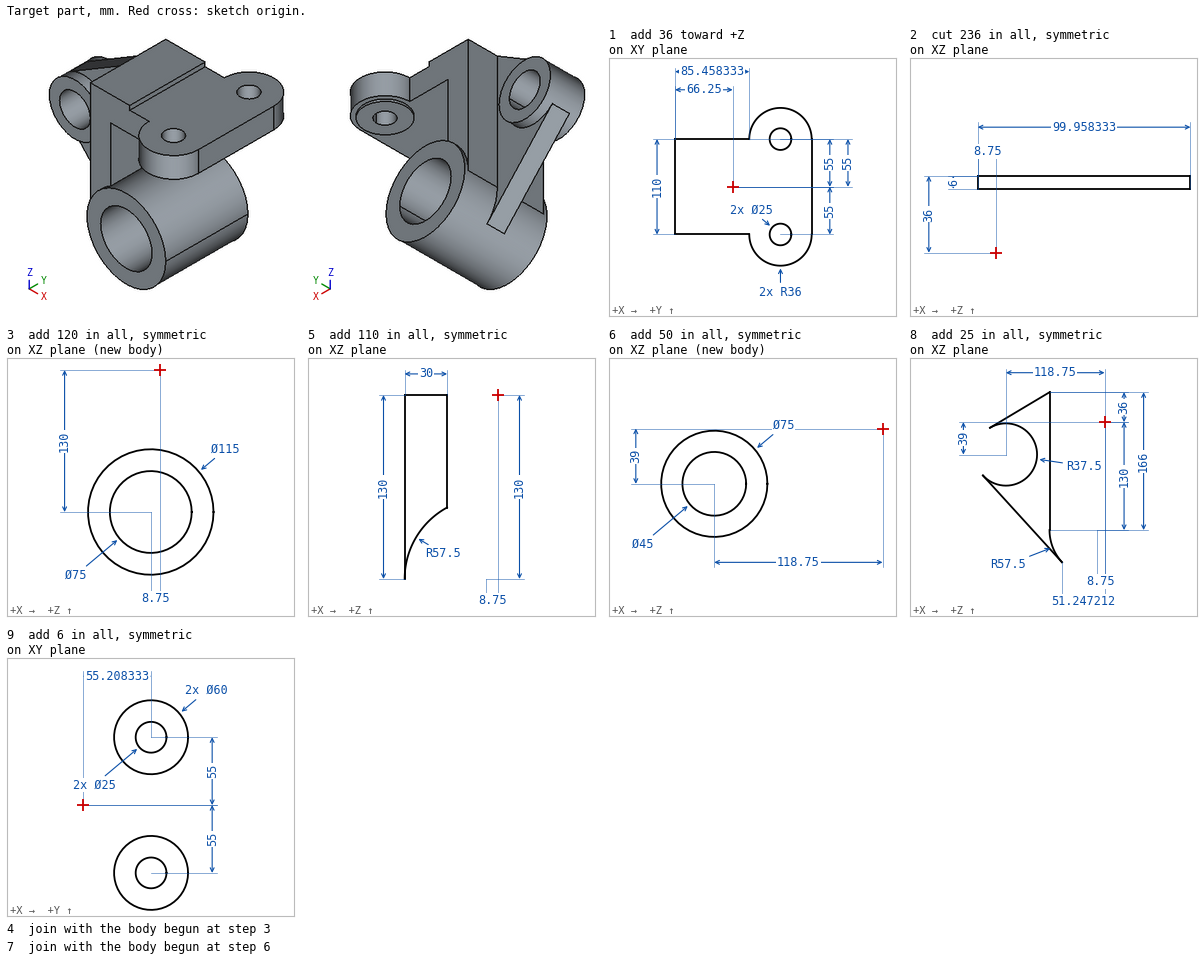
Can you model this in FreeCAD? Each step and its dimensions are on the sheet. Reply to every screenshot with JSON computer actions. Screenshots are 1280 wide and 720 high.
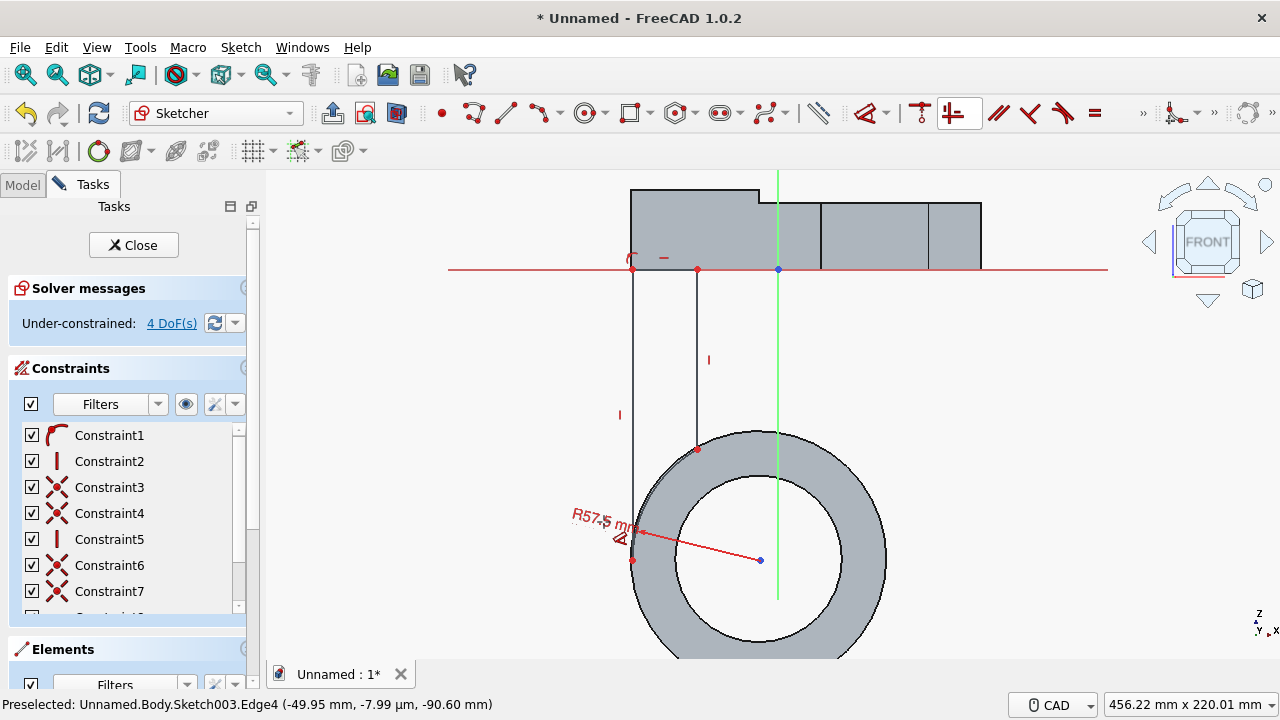
{"action": "left_click", "coordinate": [652, 270]}
{"action": "left_click", "coordinate": [665, 236]}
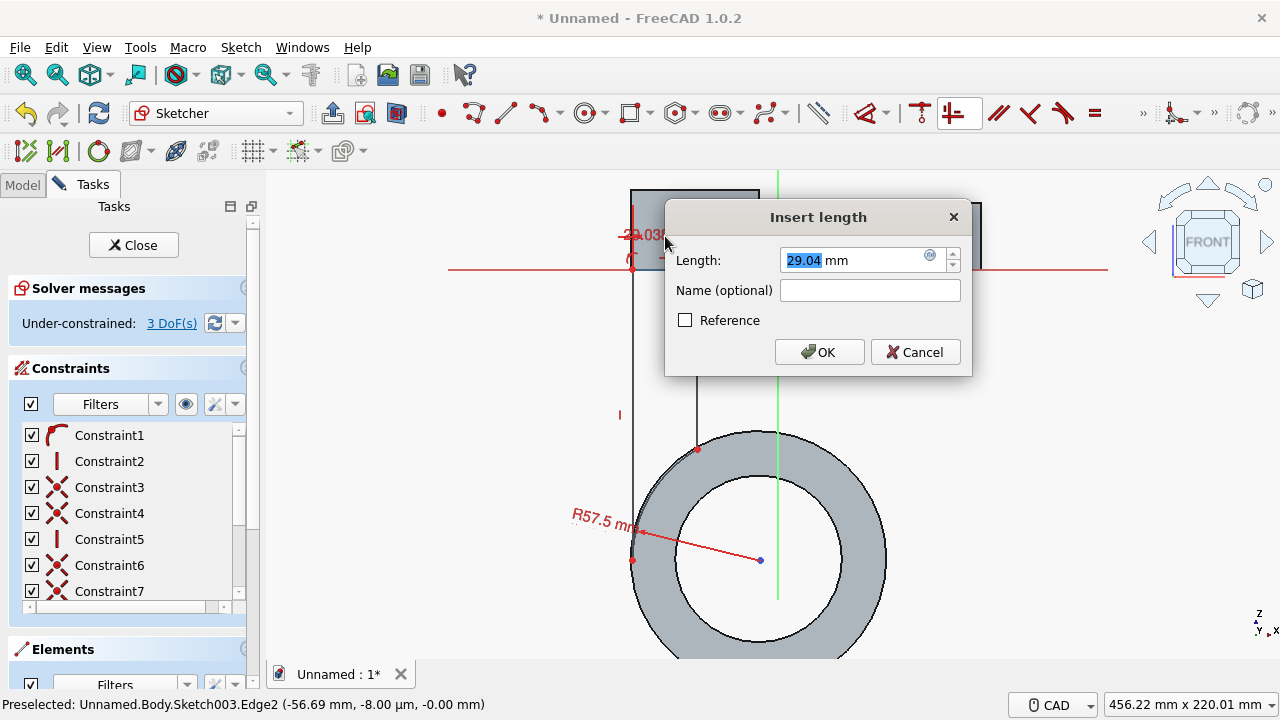
{"action": "type", "text": "30"}
{"action": "key", "text": "Return"}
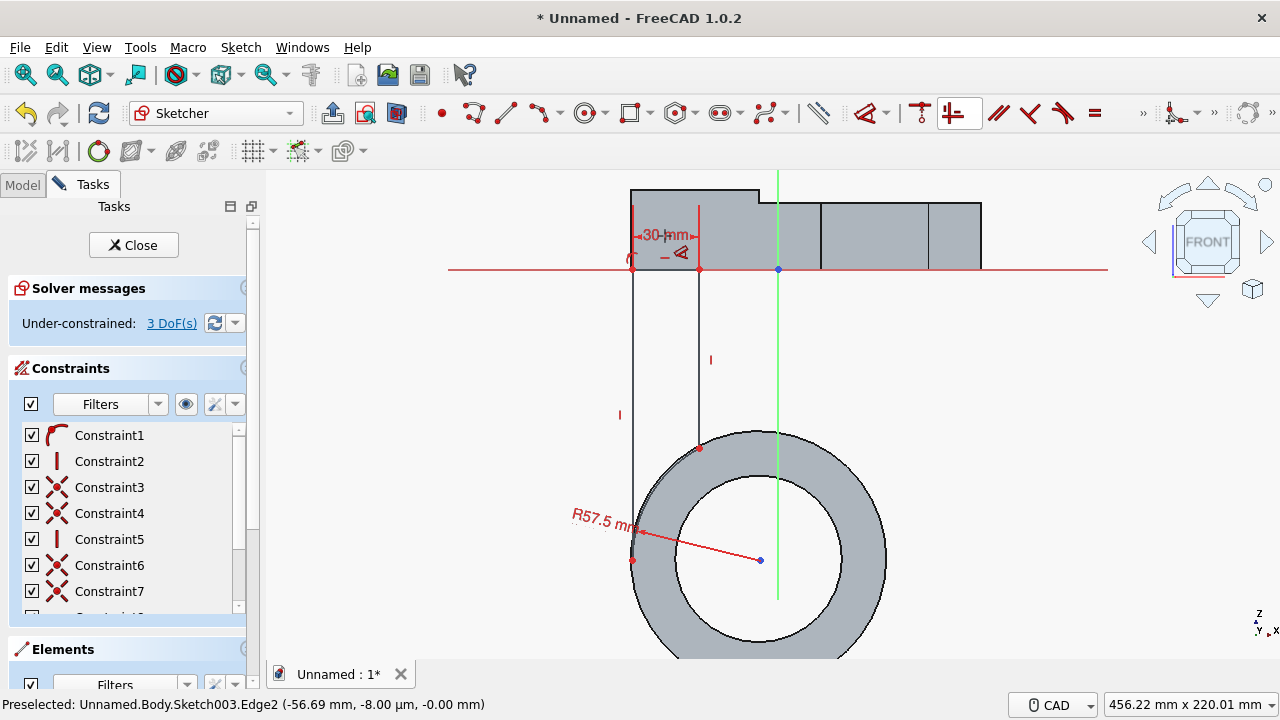
{"action": "left_click", "coordinate": [633, 473]}
{"action": "left_click", "coordinate": [599, 415]}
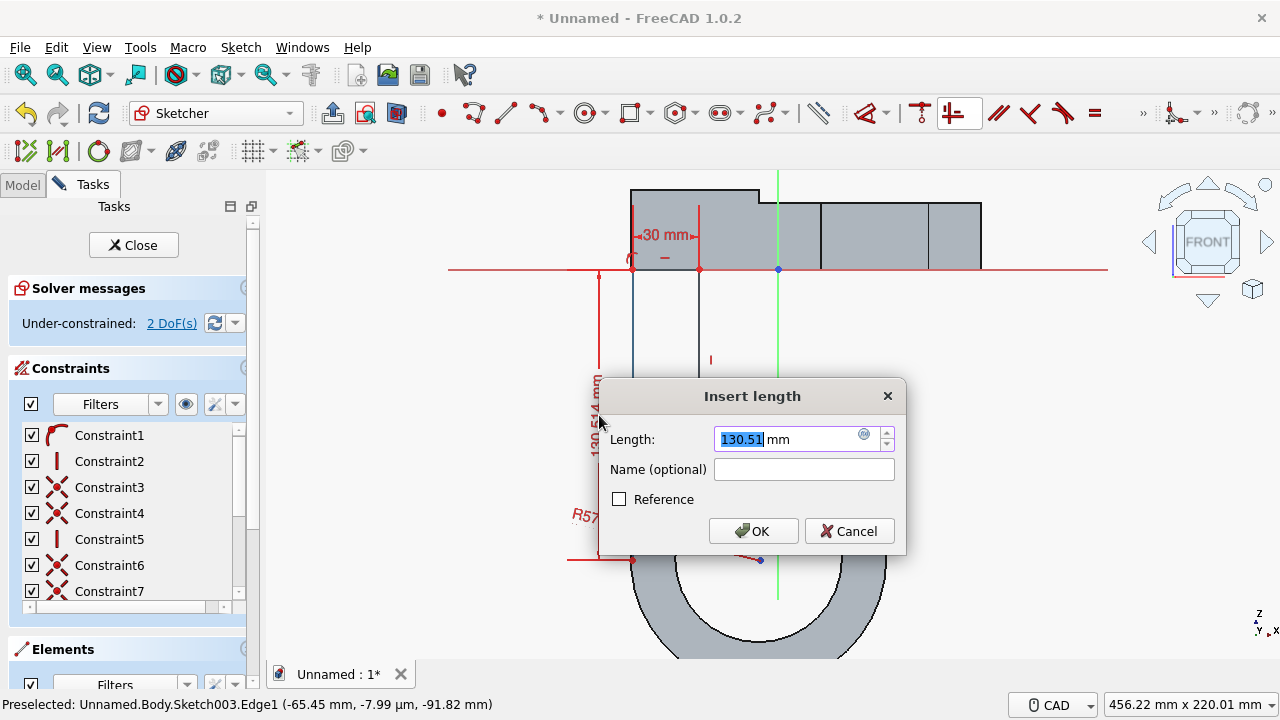
{"action": "type", "text": "130"}
{"action": "key", "text": "Return"}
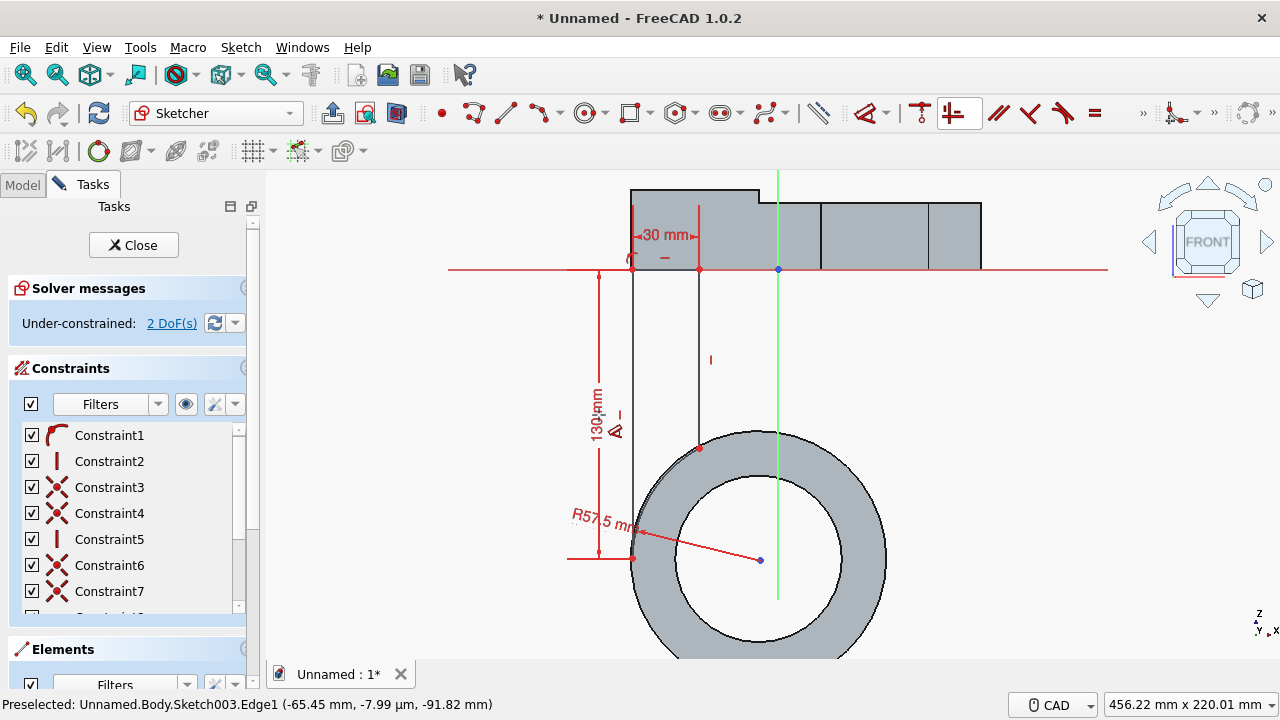
{"action": "left_click", "coordinate": [760, 561]}
{"action": "left_click", "coordinate": [812, 415]}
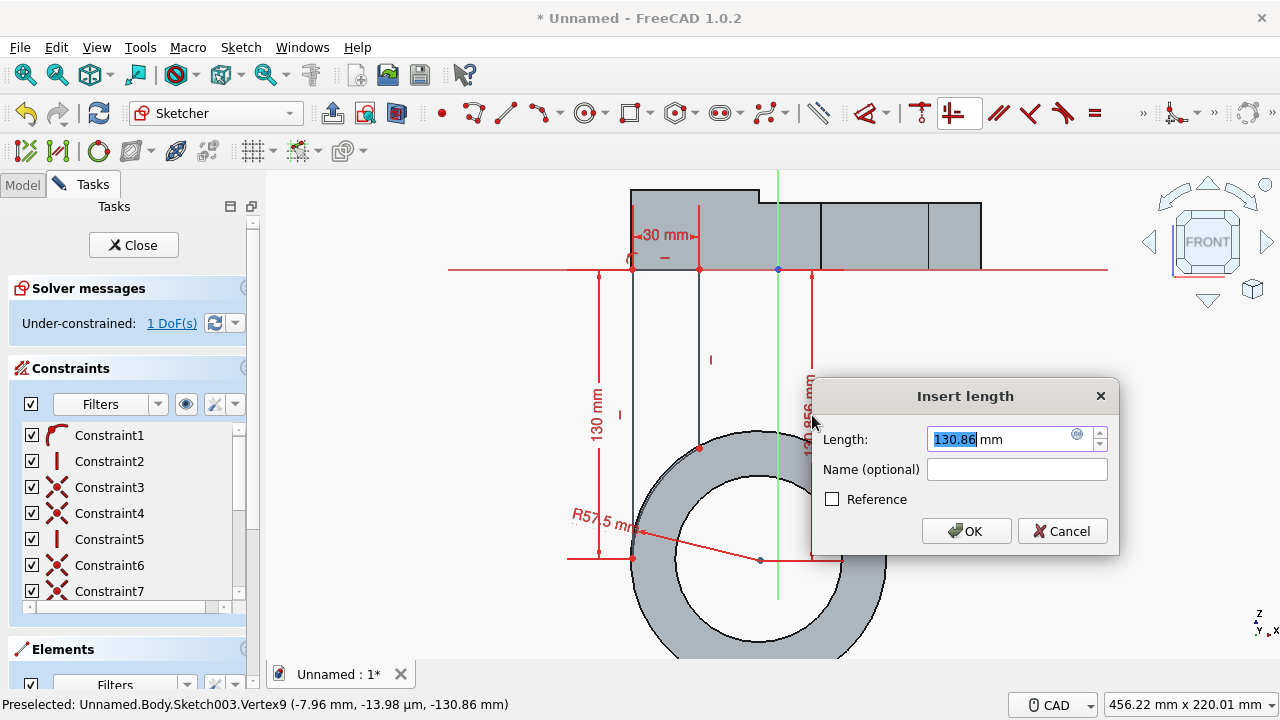
{"action": "type", "text": "130"}
{"action": "key", "text": "Return"}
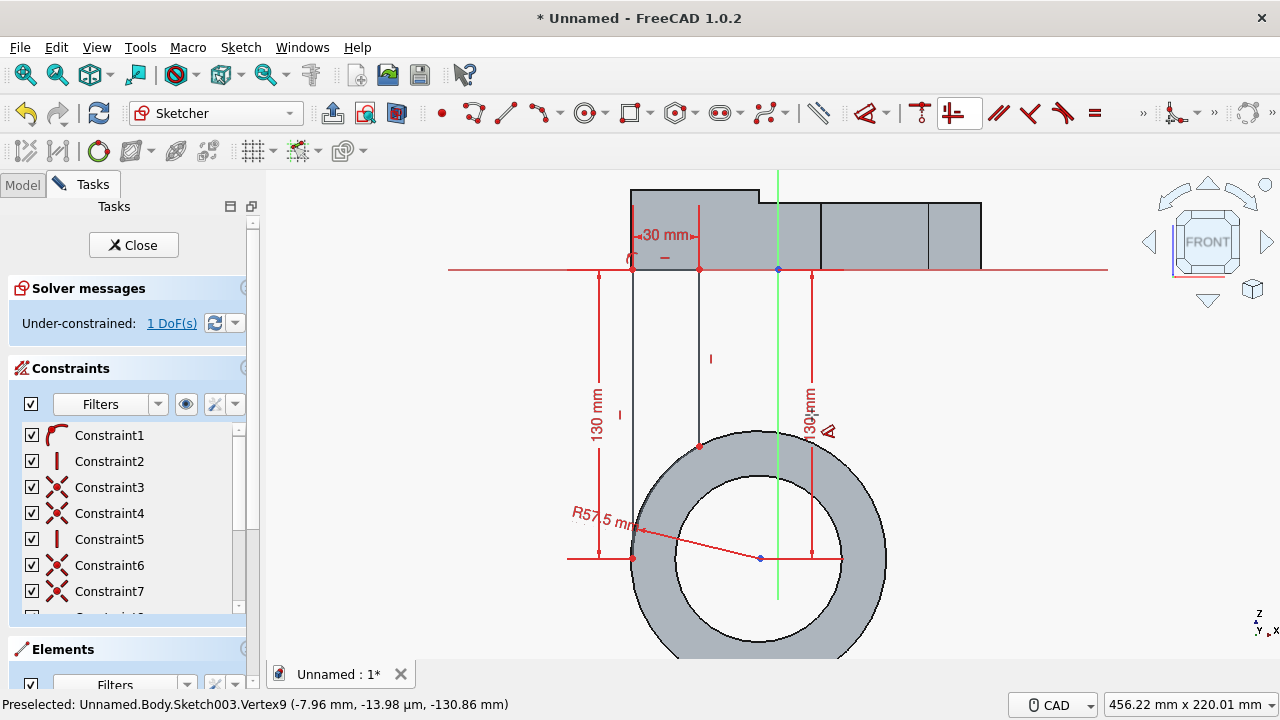
{"action": "scroll", "coordinate": [760, 559], "scroll_direction": "up", "scroll_amount": 4}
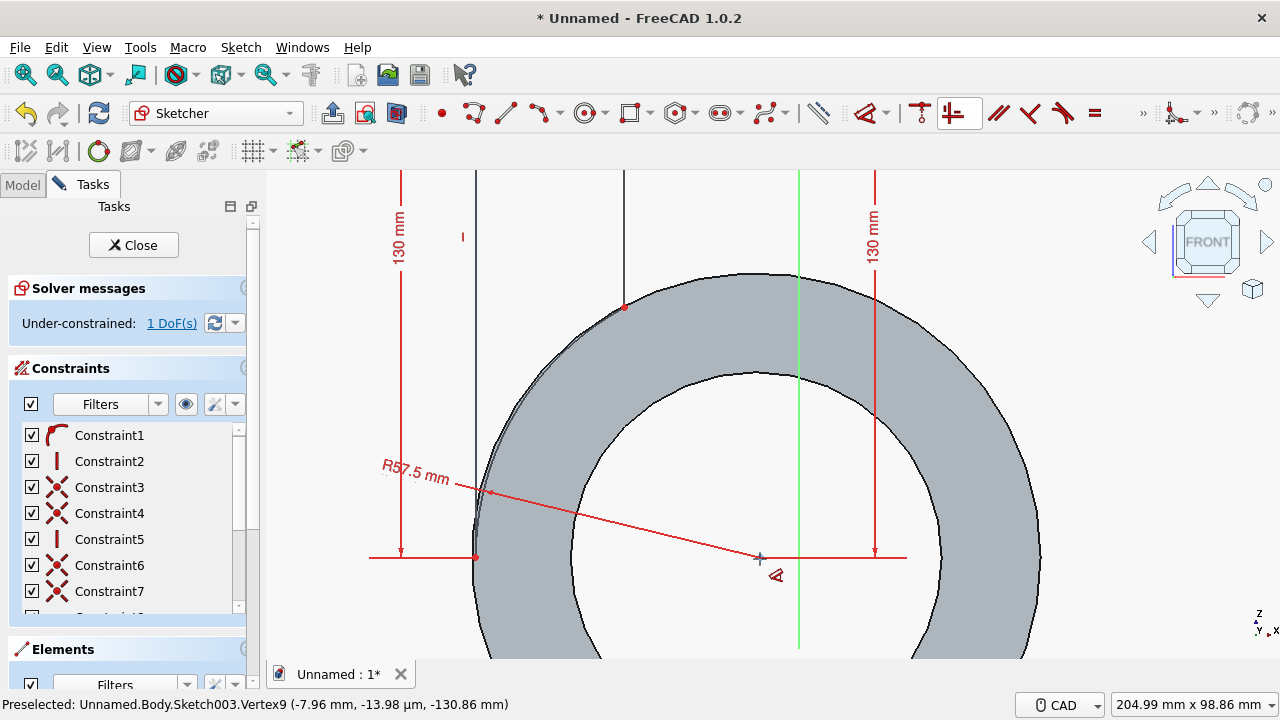
{"action": "left_click", "coordinate": [760, 558]}
{"action": "left_click", "coordinate": [780, 592]}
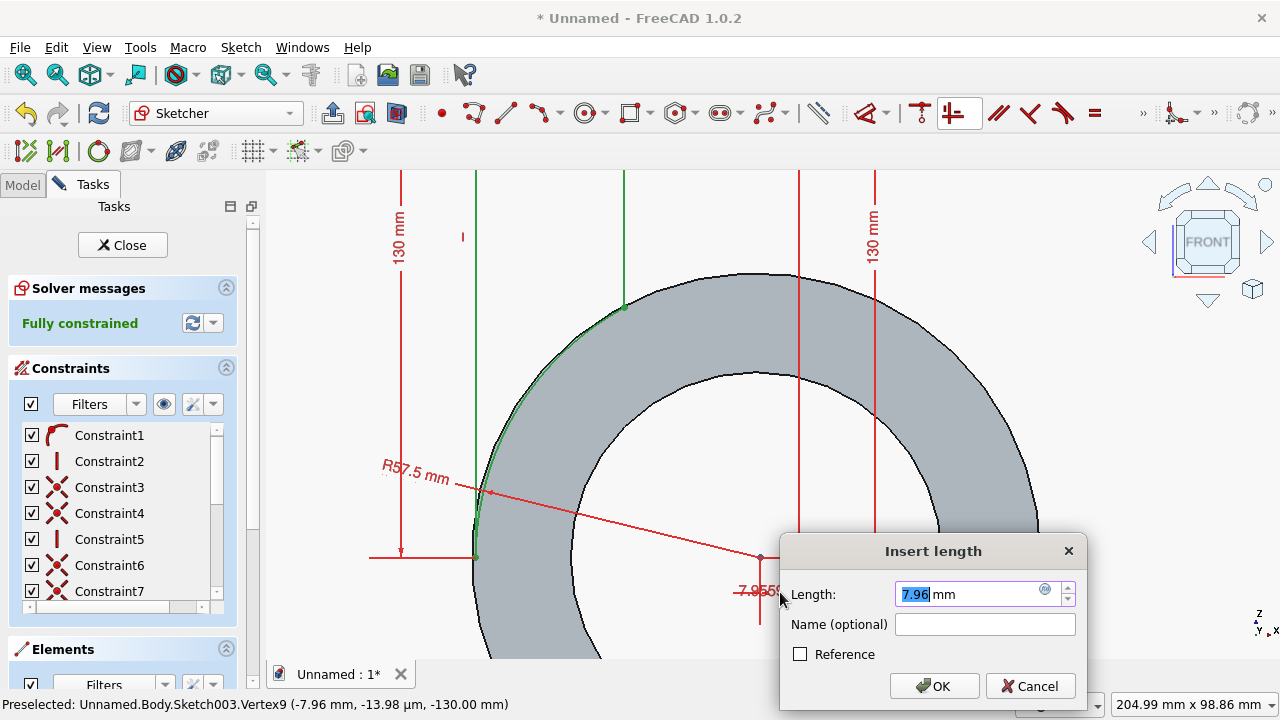
{"action": "type", "text": "8.75"}
{"action": "key", "text": "Return"}
{"action": "key", "text": "Escape"}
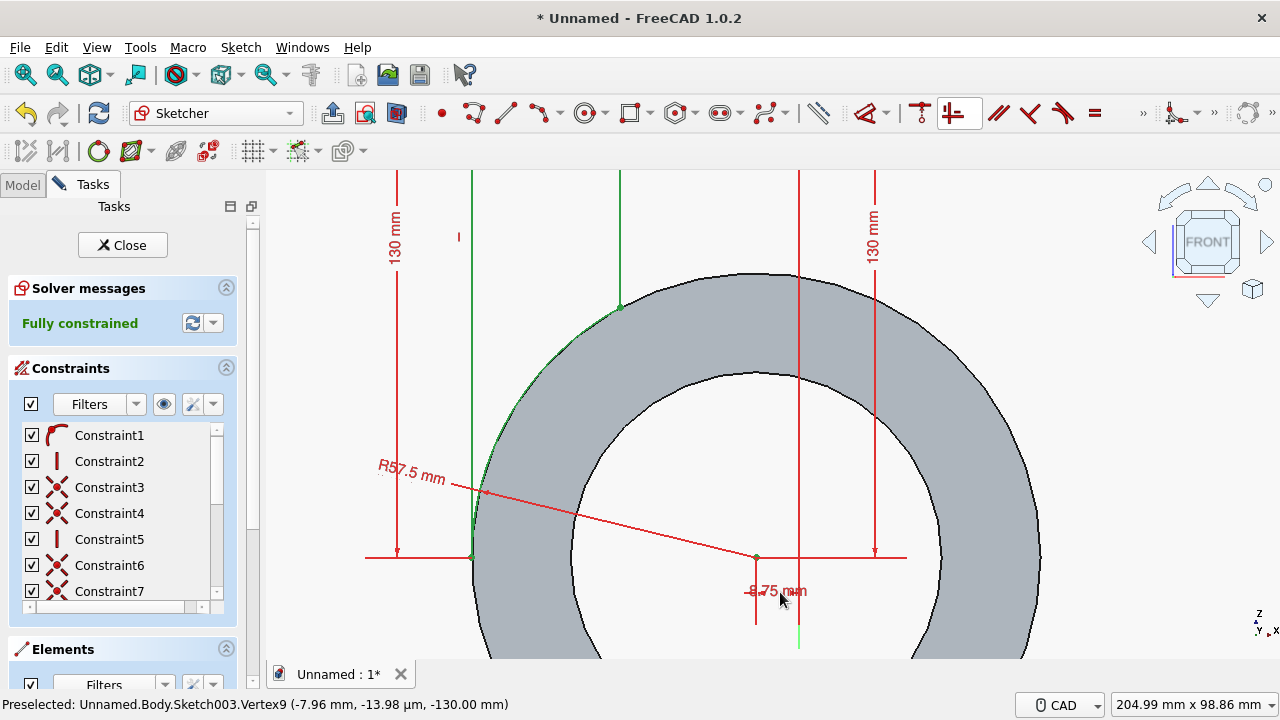
{"action": "left_click", "coordinate": [123, 245]}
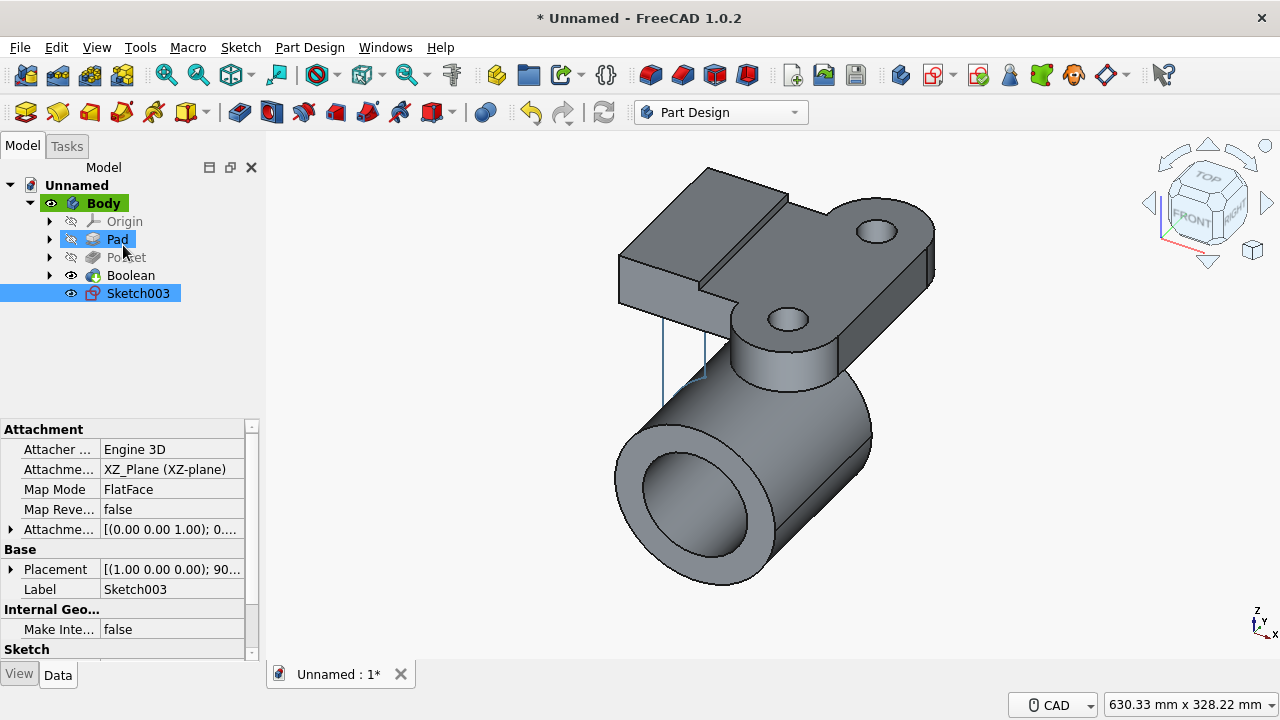
{"action": "left_click", "coordinate": [26, 112]}